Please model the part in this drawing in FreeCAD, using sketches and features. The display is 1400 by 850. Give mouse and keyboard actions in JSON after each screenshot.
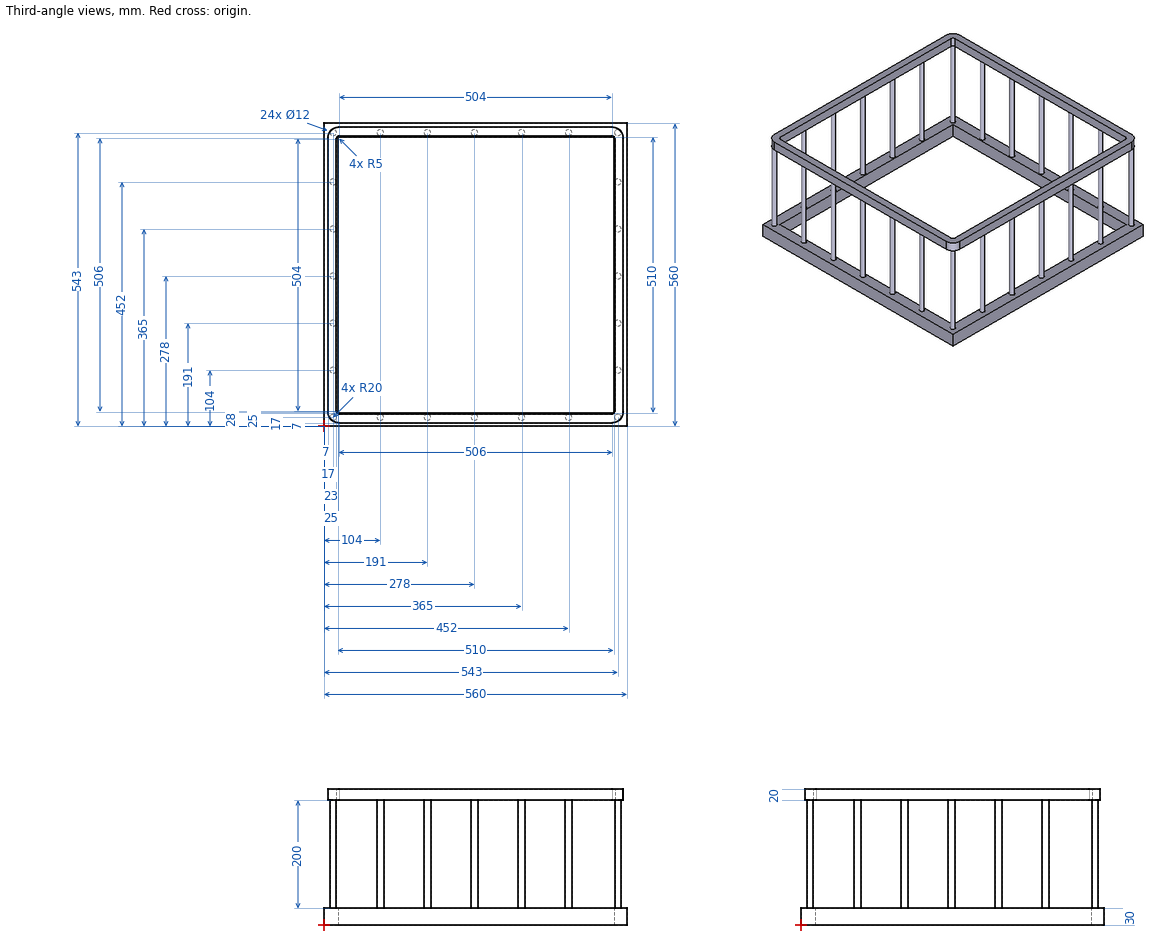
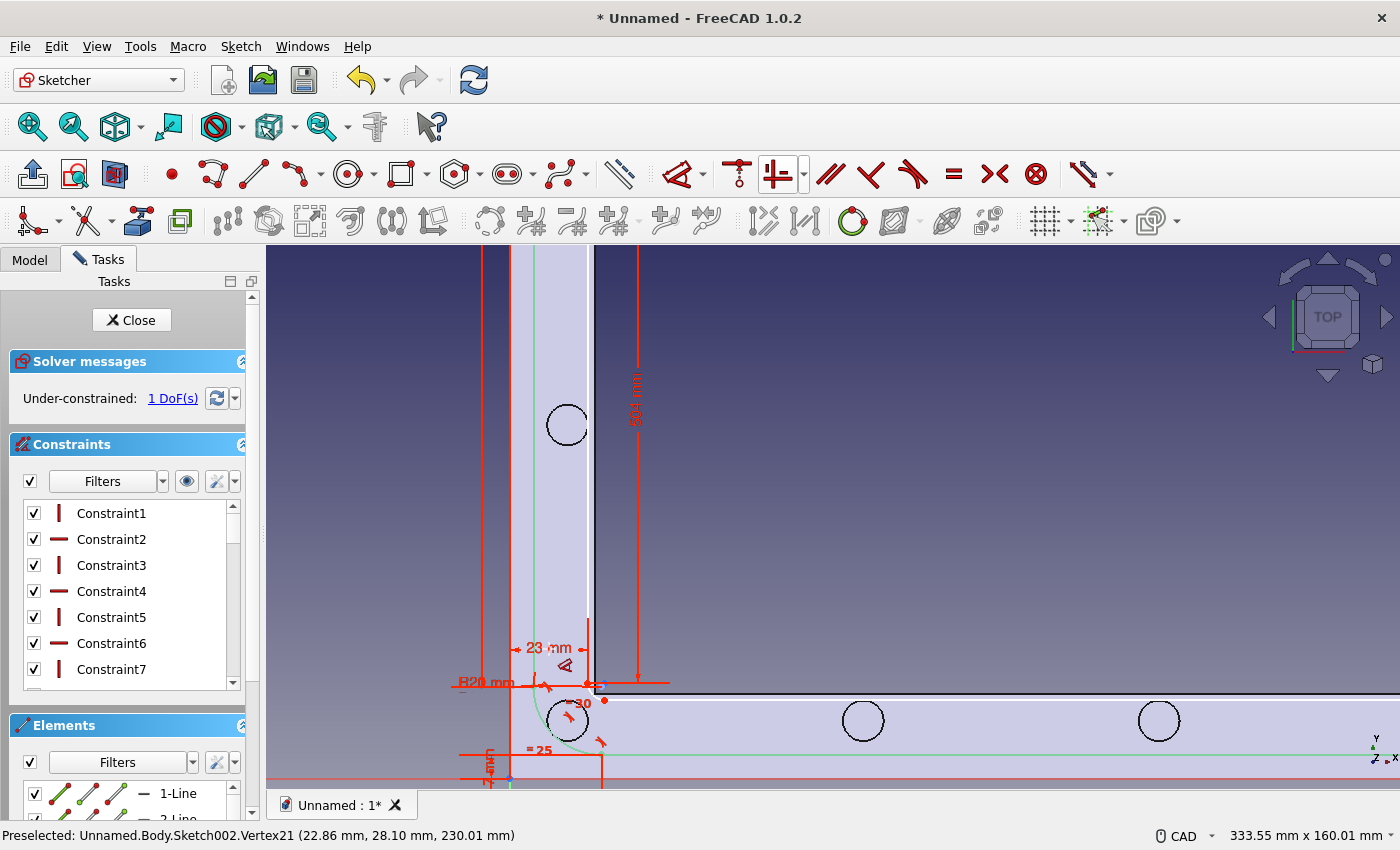
{"action": "left_click", "coordinate": [588, 683]}
{"action": "left_click", "coordinate": [476, 722]}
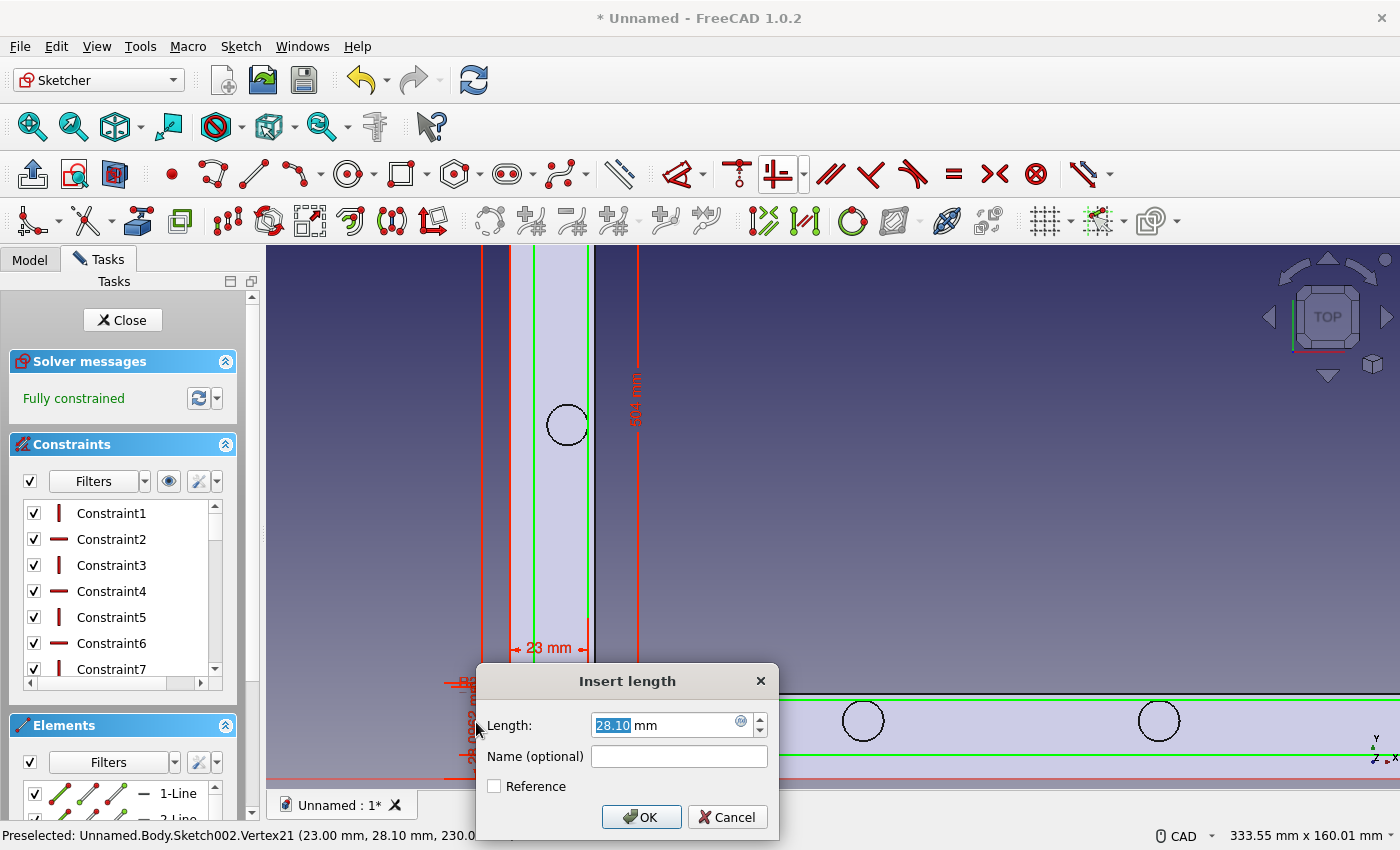
{"action": "type", "text": "28"}
{"action": "key", "text": "Return"}
{"action": "key", "text": "Escape"}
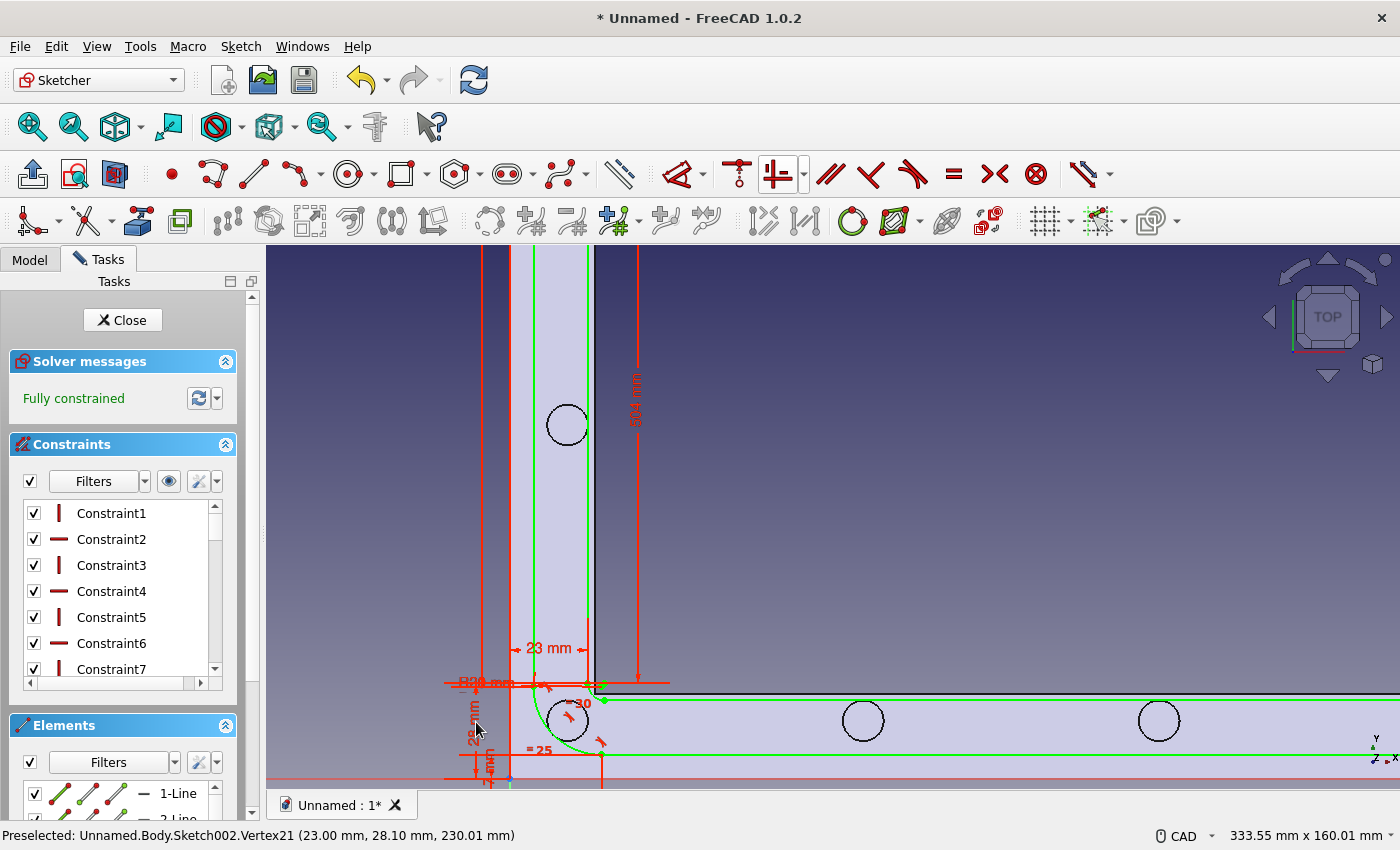
{"action": "left_click", "coordinate": [123, 320]}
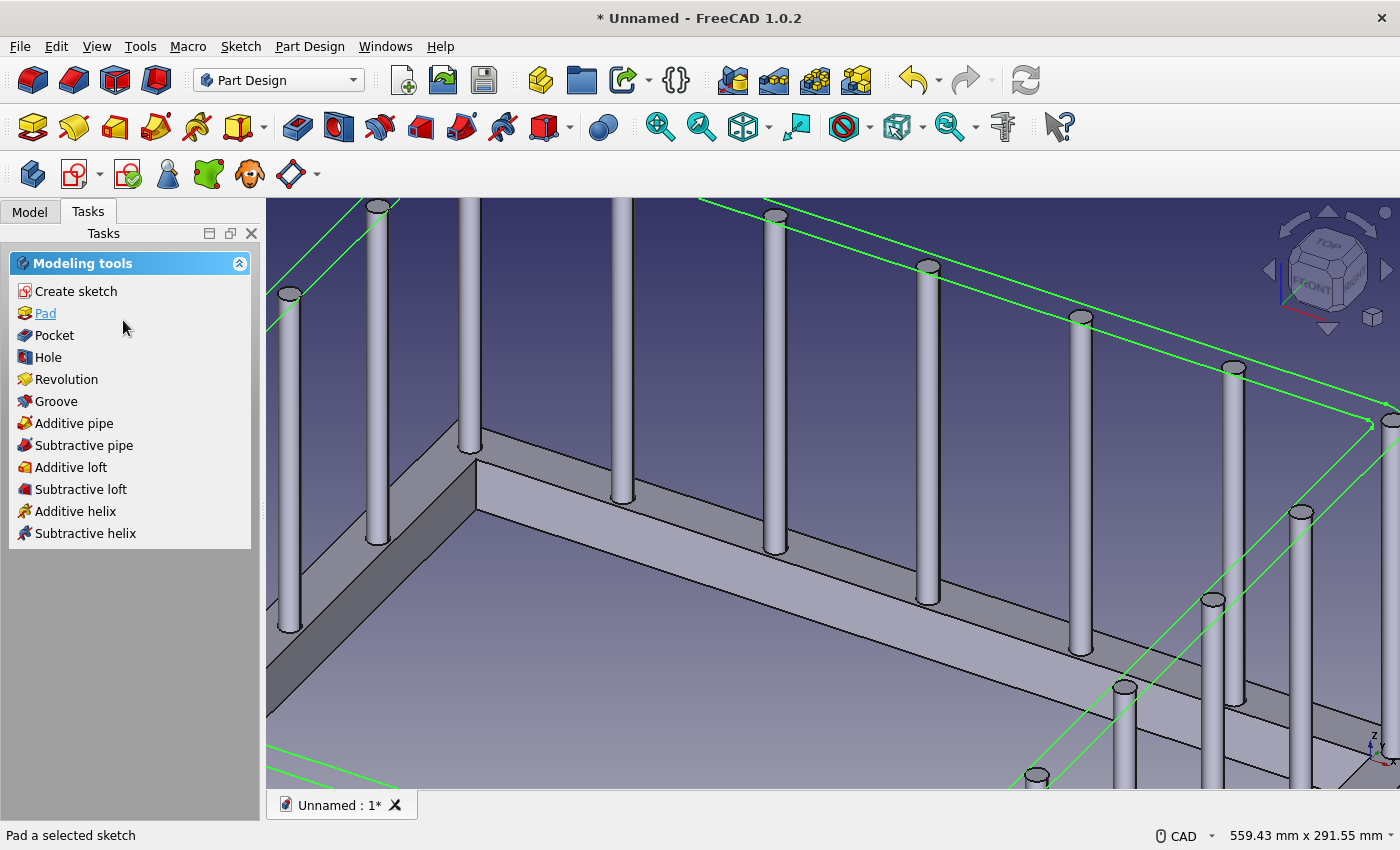
{"action": "left_click", "coordinate": [33, 128]}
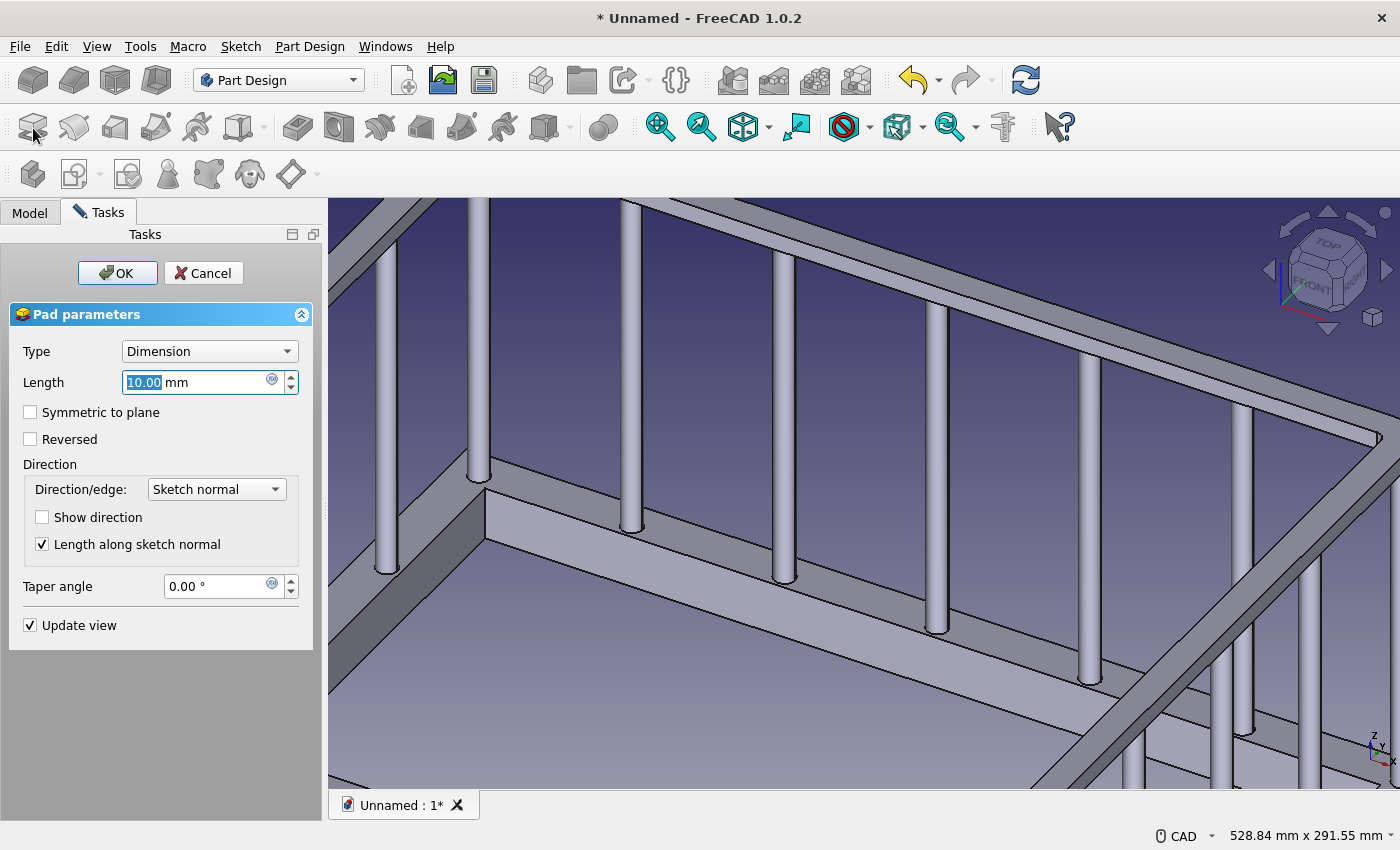
{"action": "type", "text": "20"}
{"action": "key", "text": "Tab"}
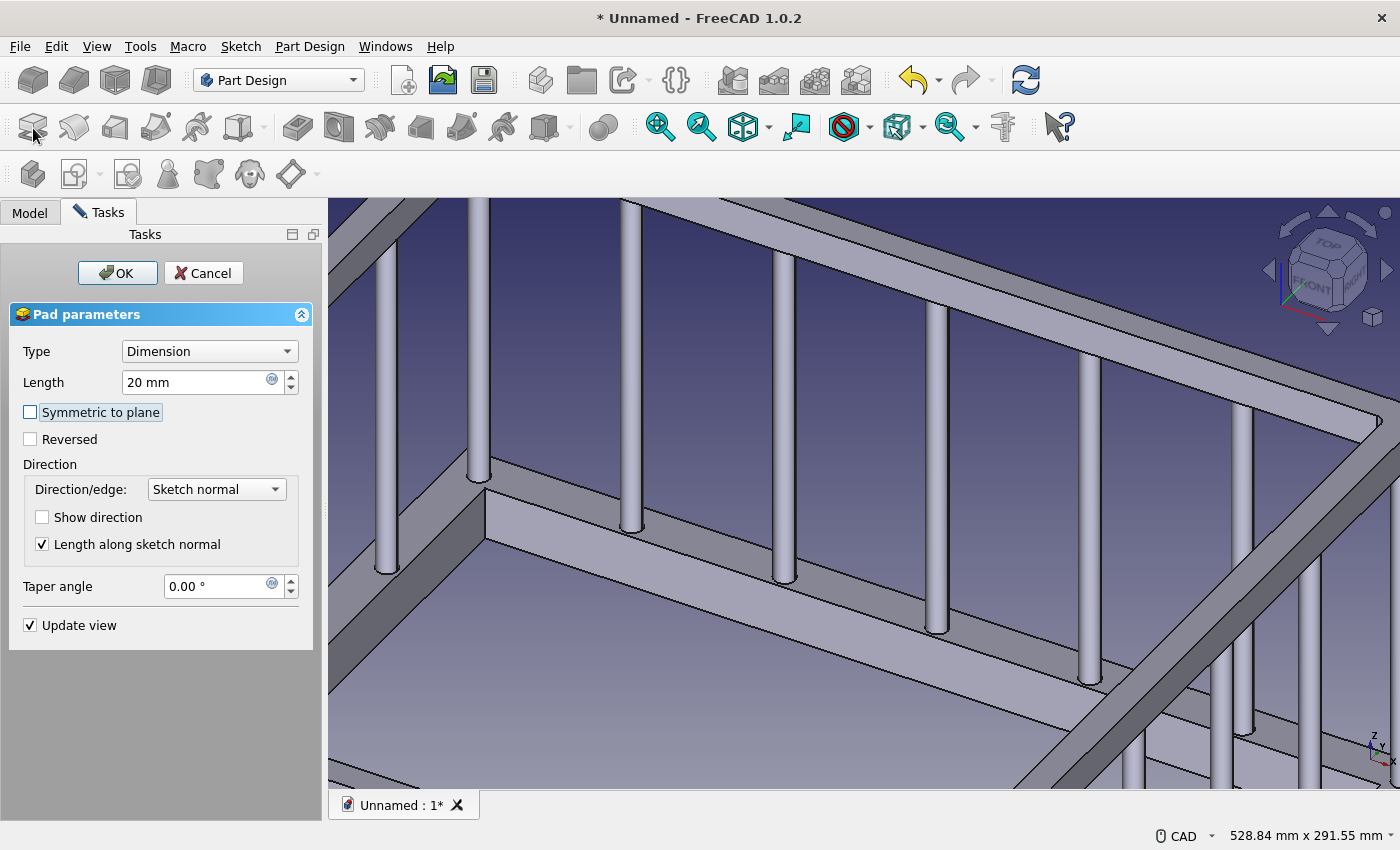
{"action": "left_click", "coordinate": [118, 273]}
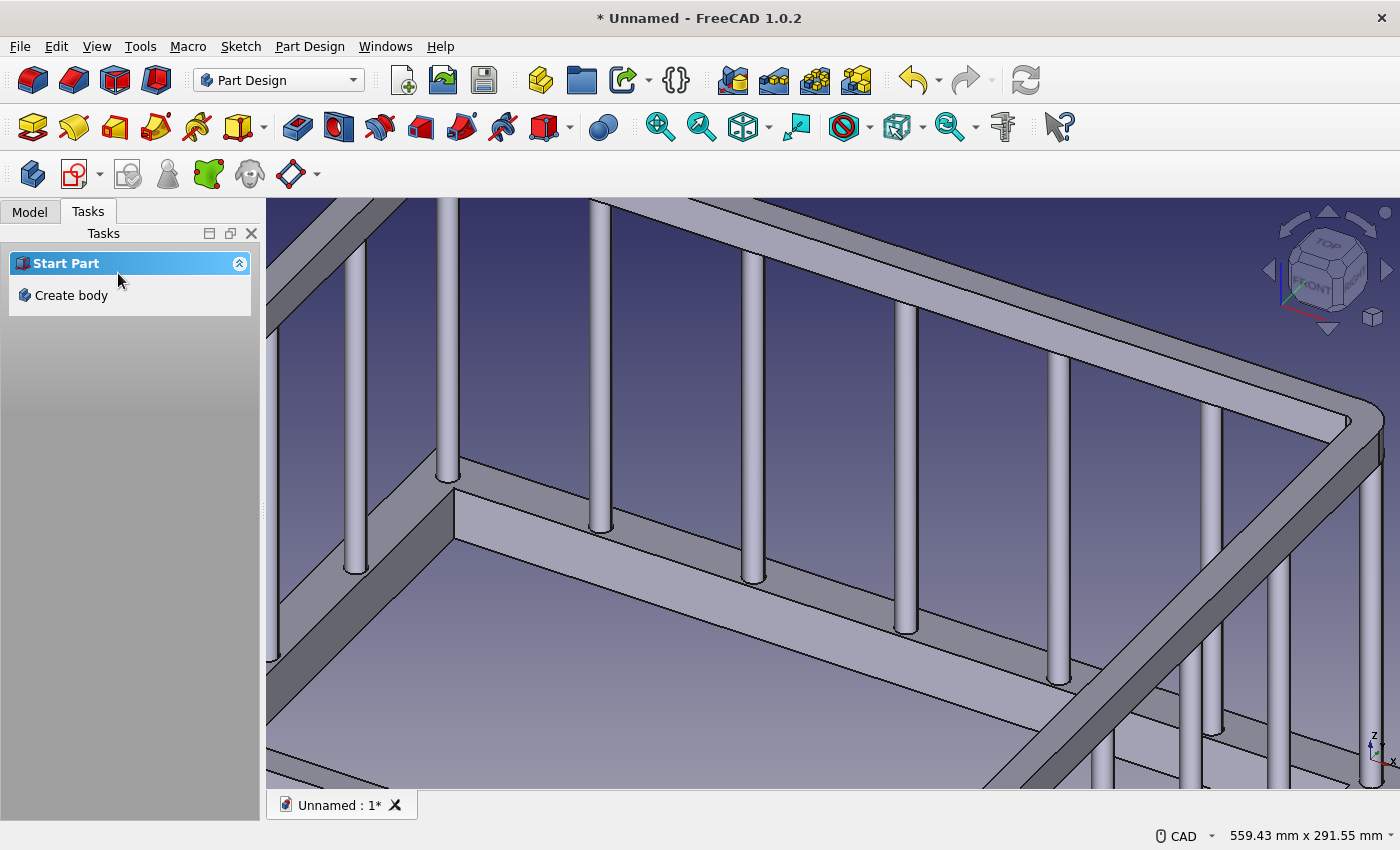
{"action": "key", "text": "0"}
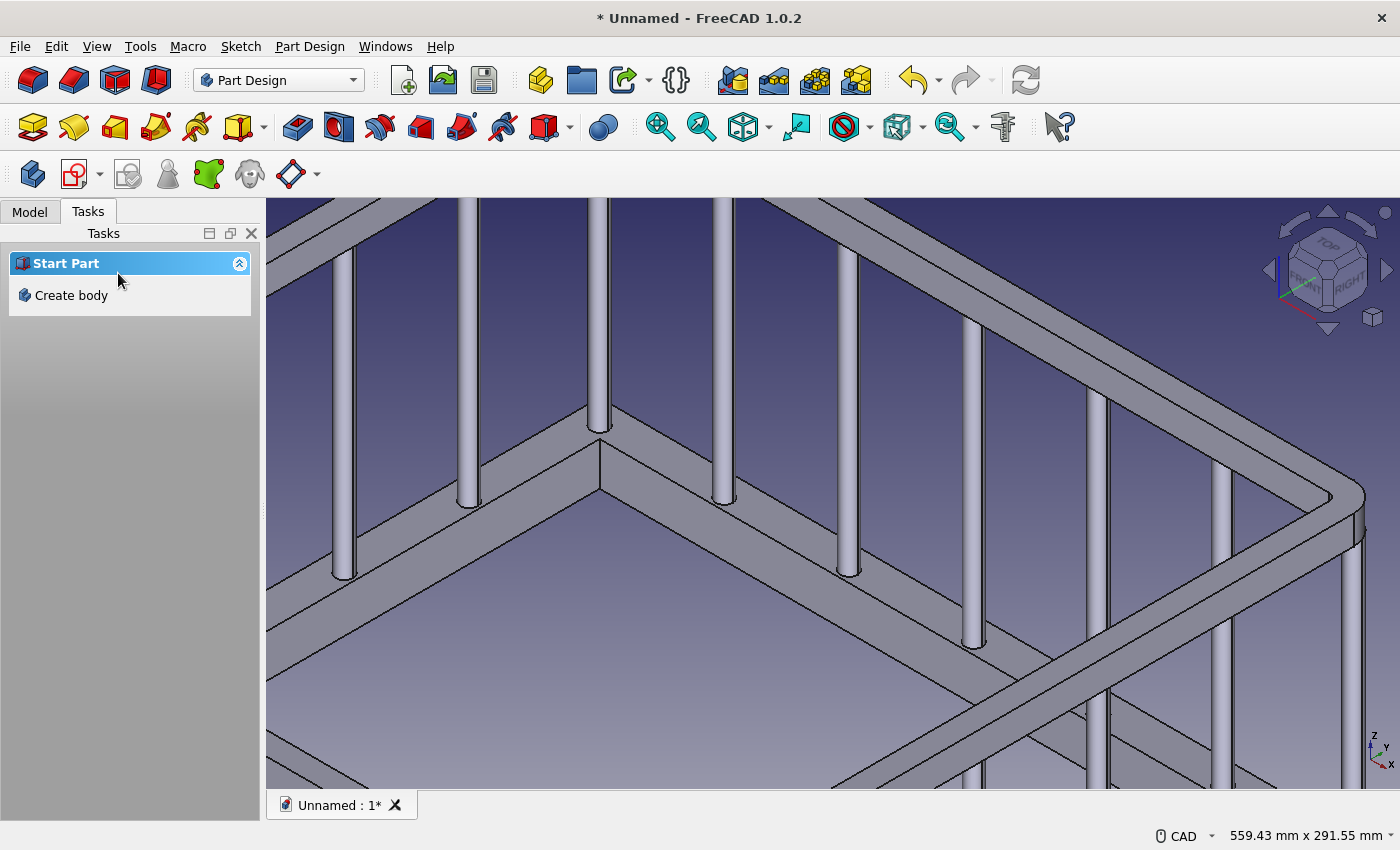
{"action": "left_click", "coordinate": [661, 128]}